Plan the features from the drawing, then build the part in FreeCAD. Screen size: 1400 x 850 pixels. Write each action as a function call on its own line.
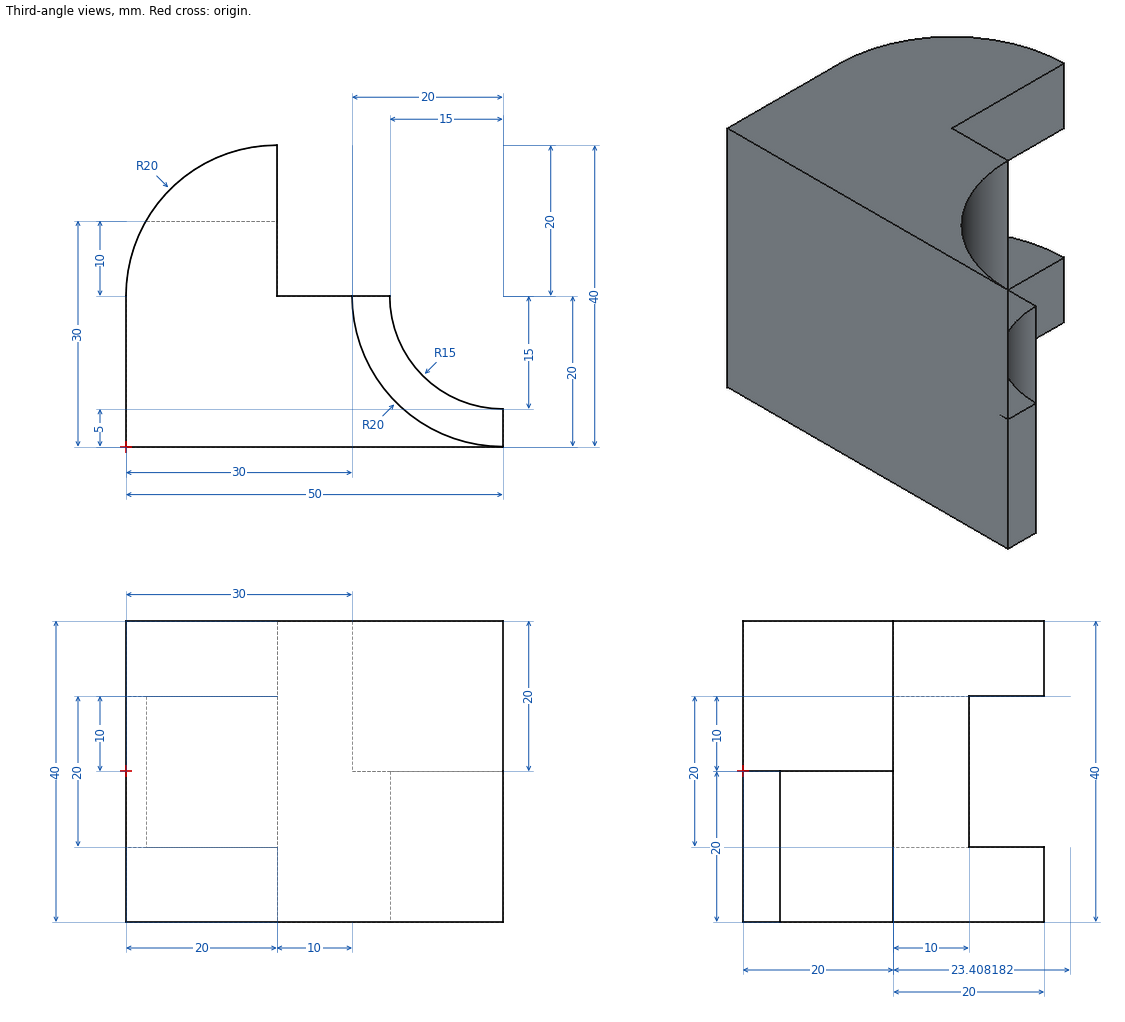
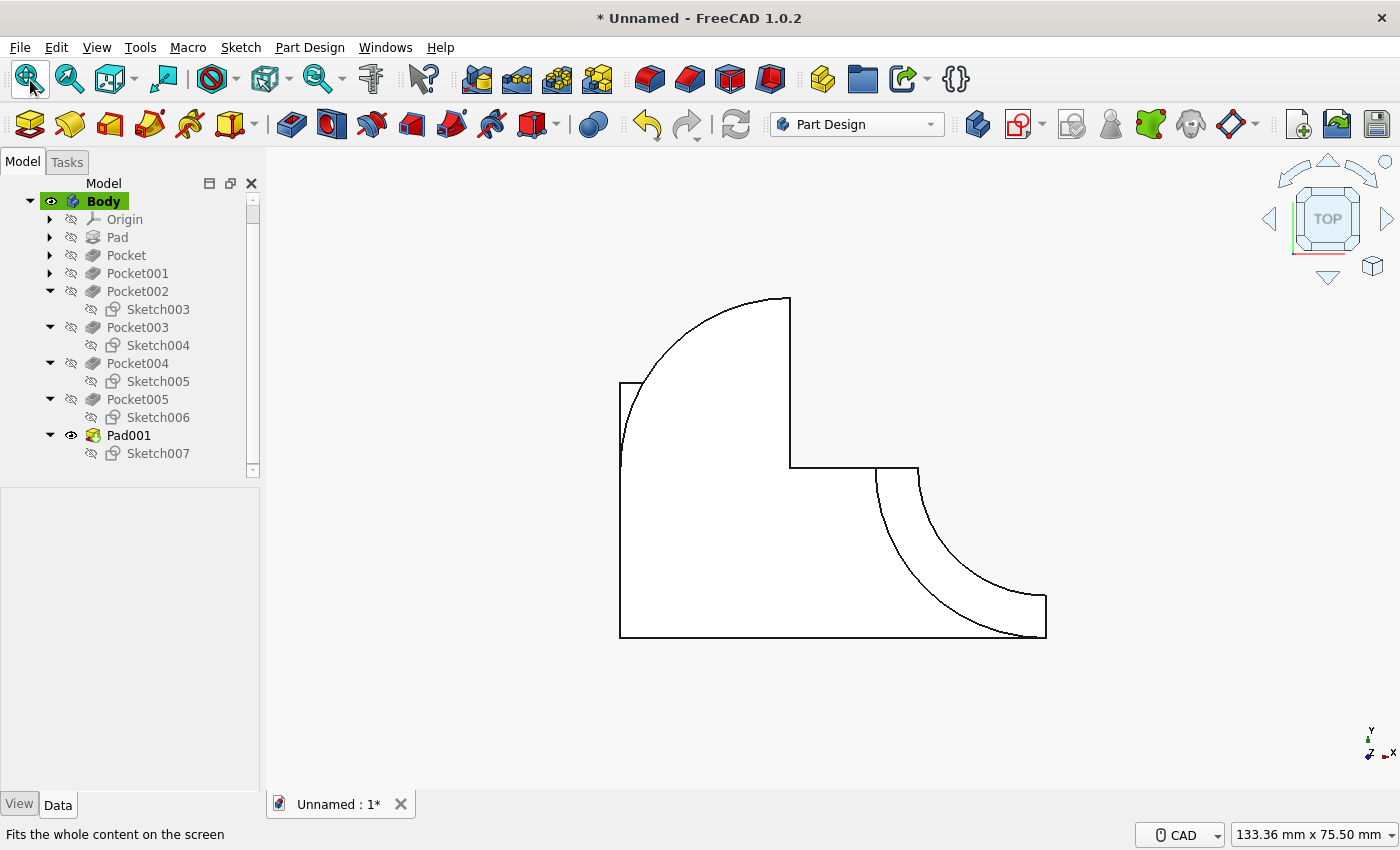
scroll(632, 388, up, 4)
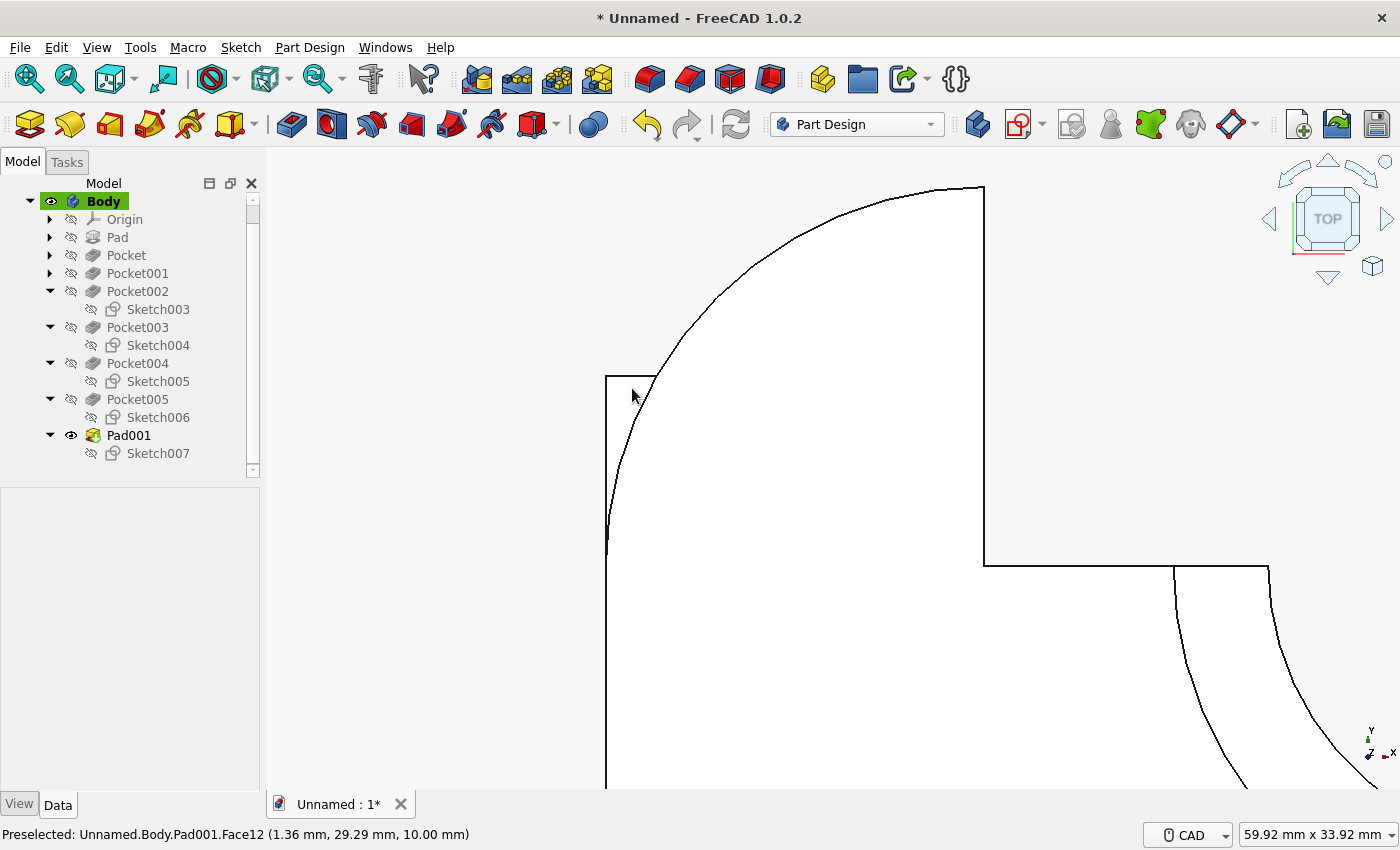
click(631, 389)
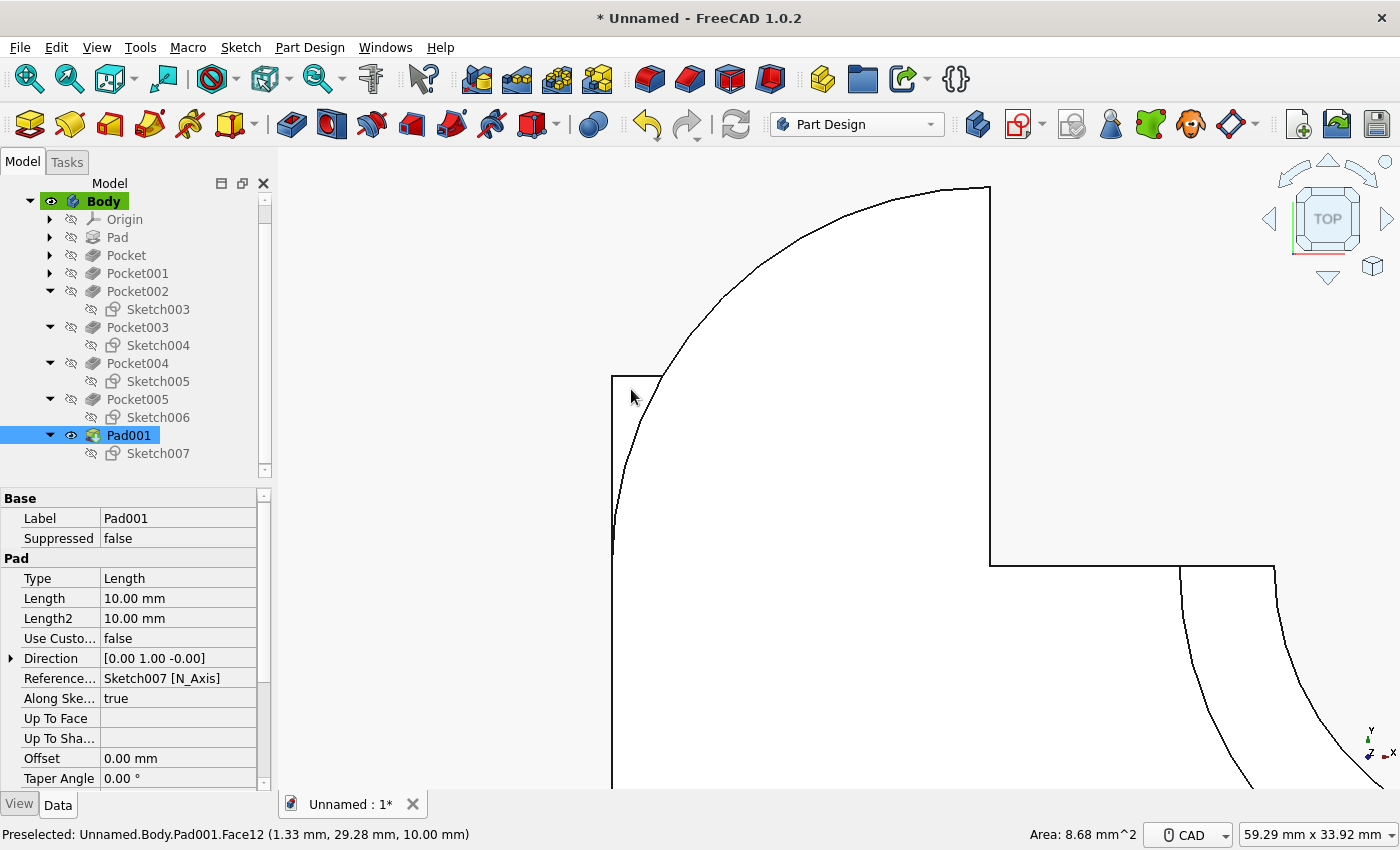
click(1018, 124)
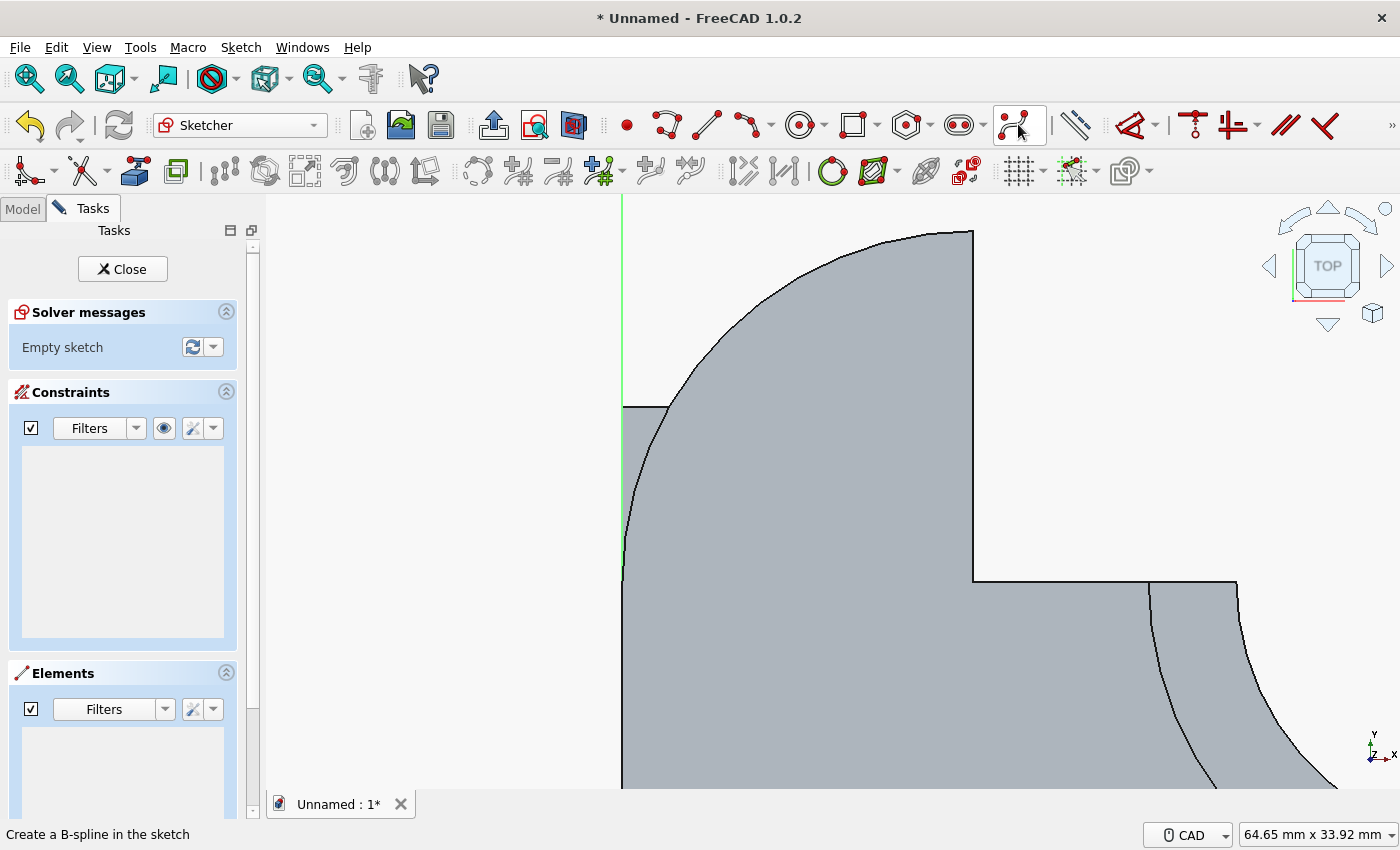
scroll(549, 496, up, 4)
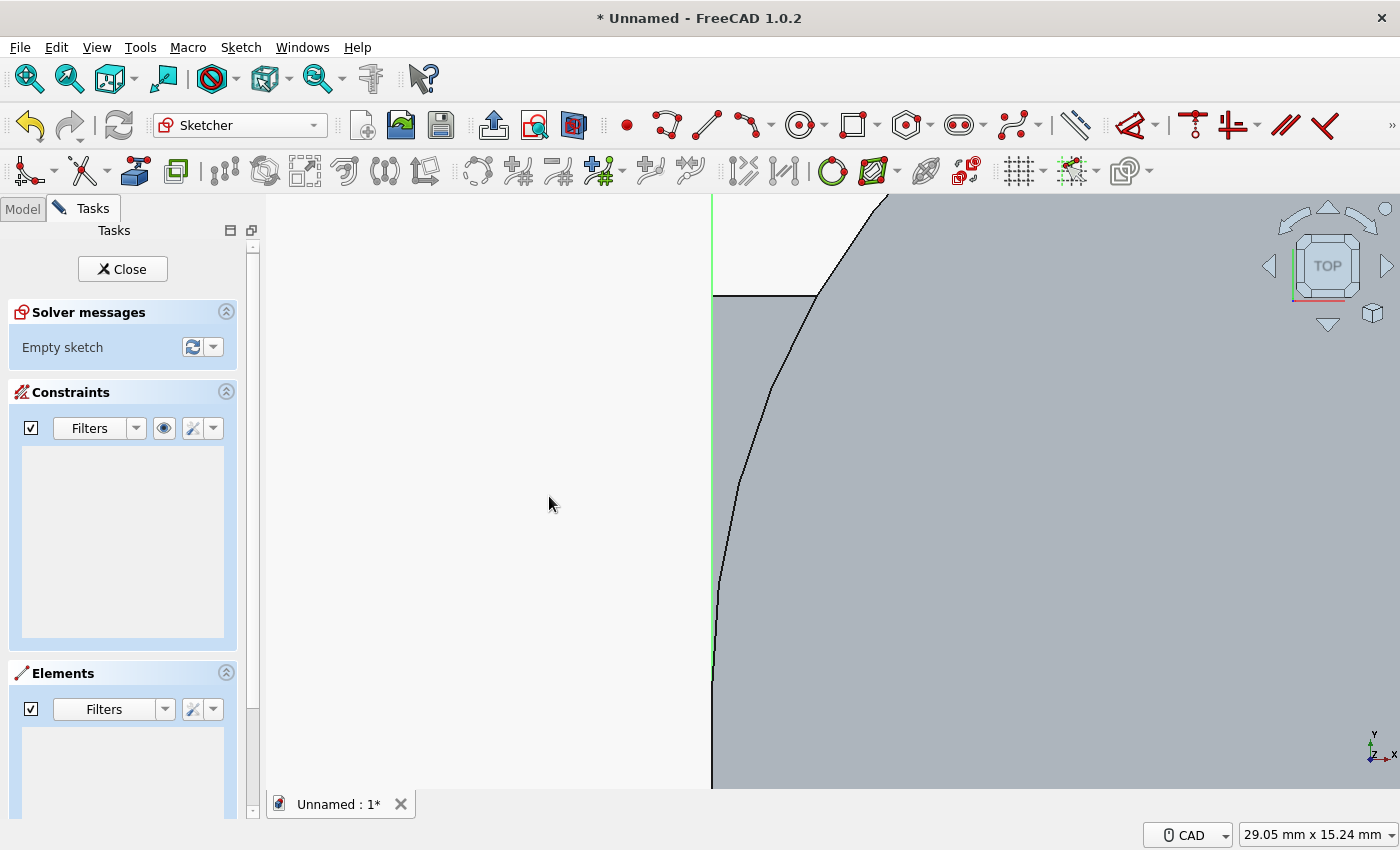
click(668, 126)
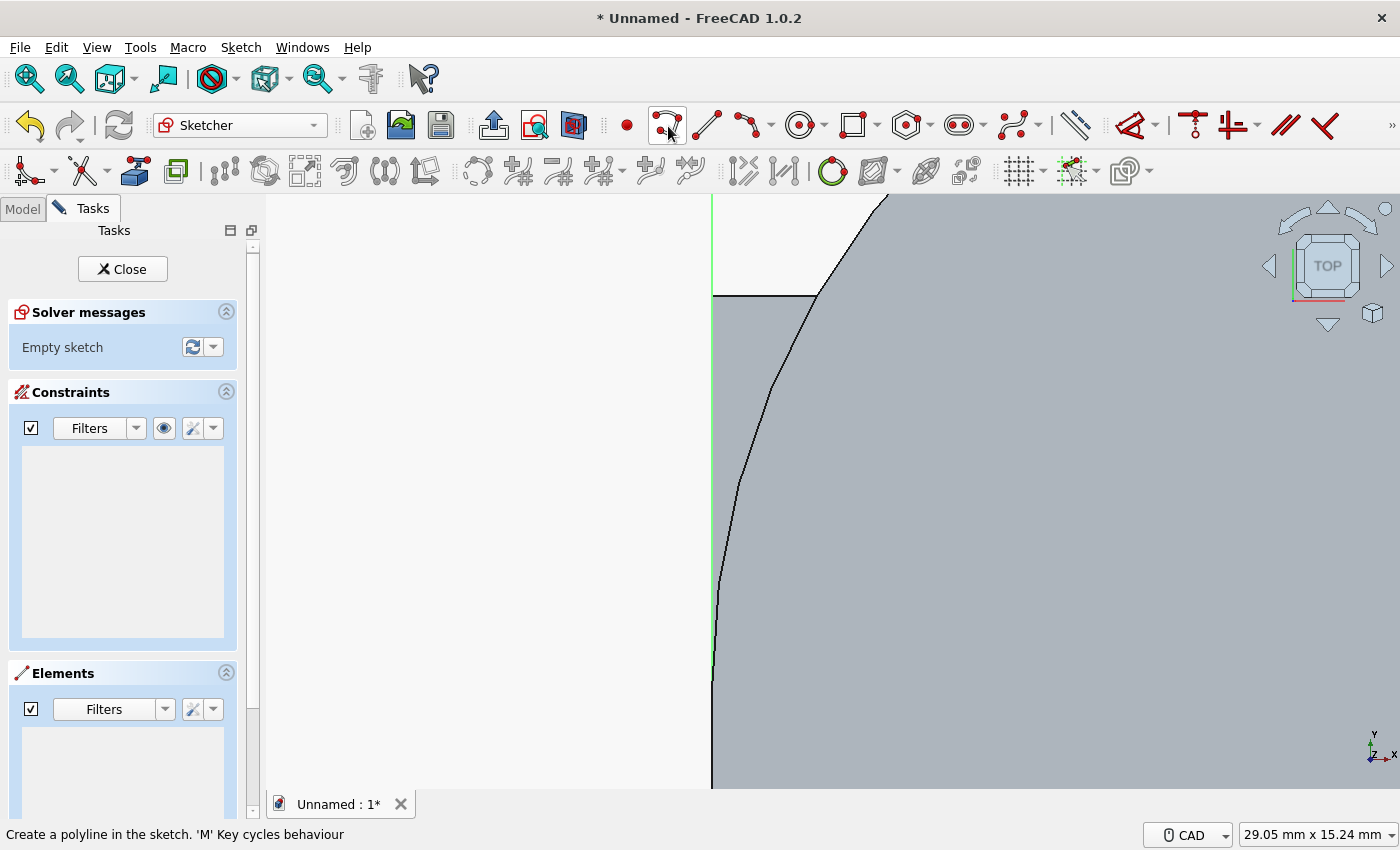
click(817, 296)
click(712, 296)
click(721, 687)
right_click(721, 687)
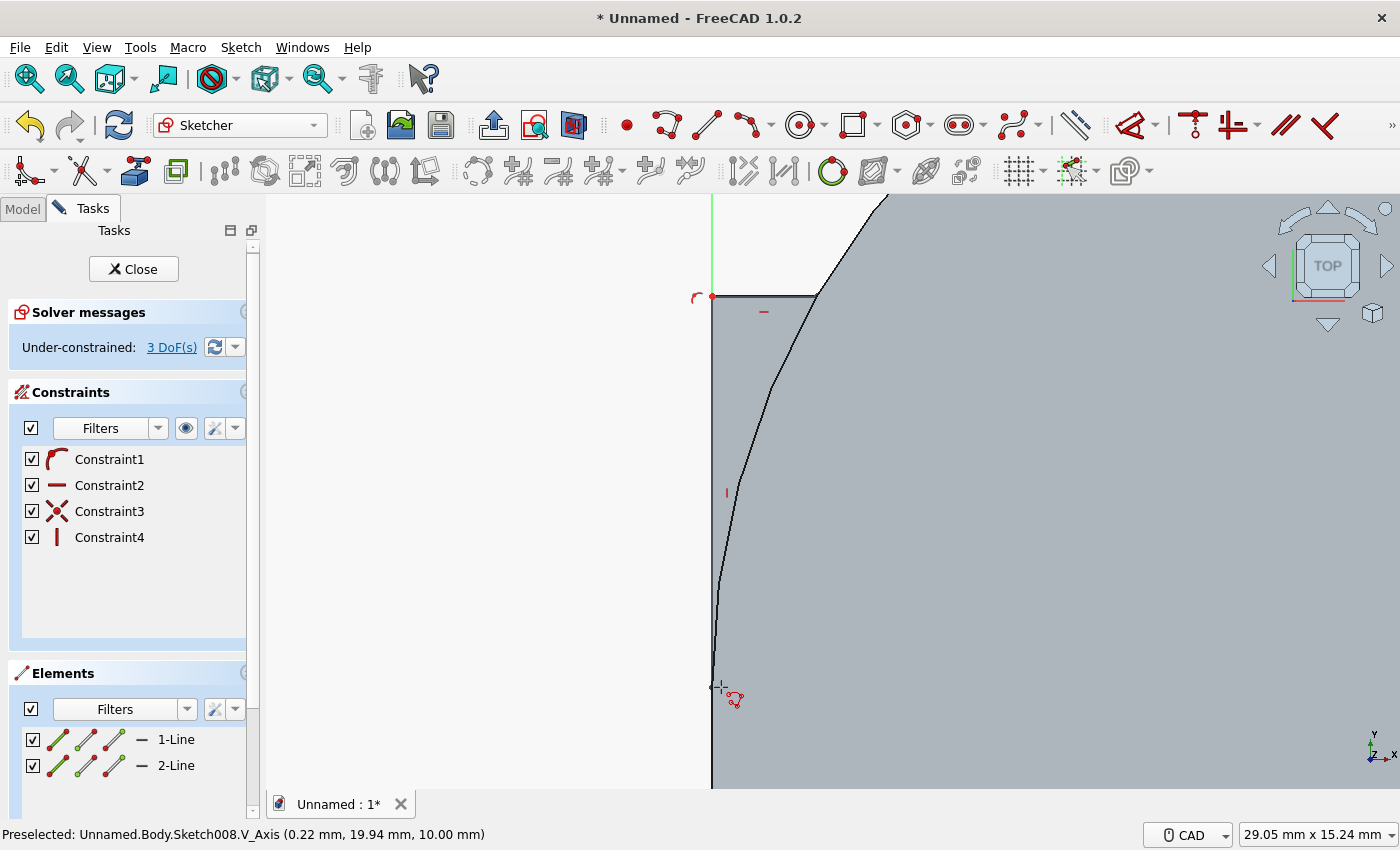
click(748, 126)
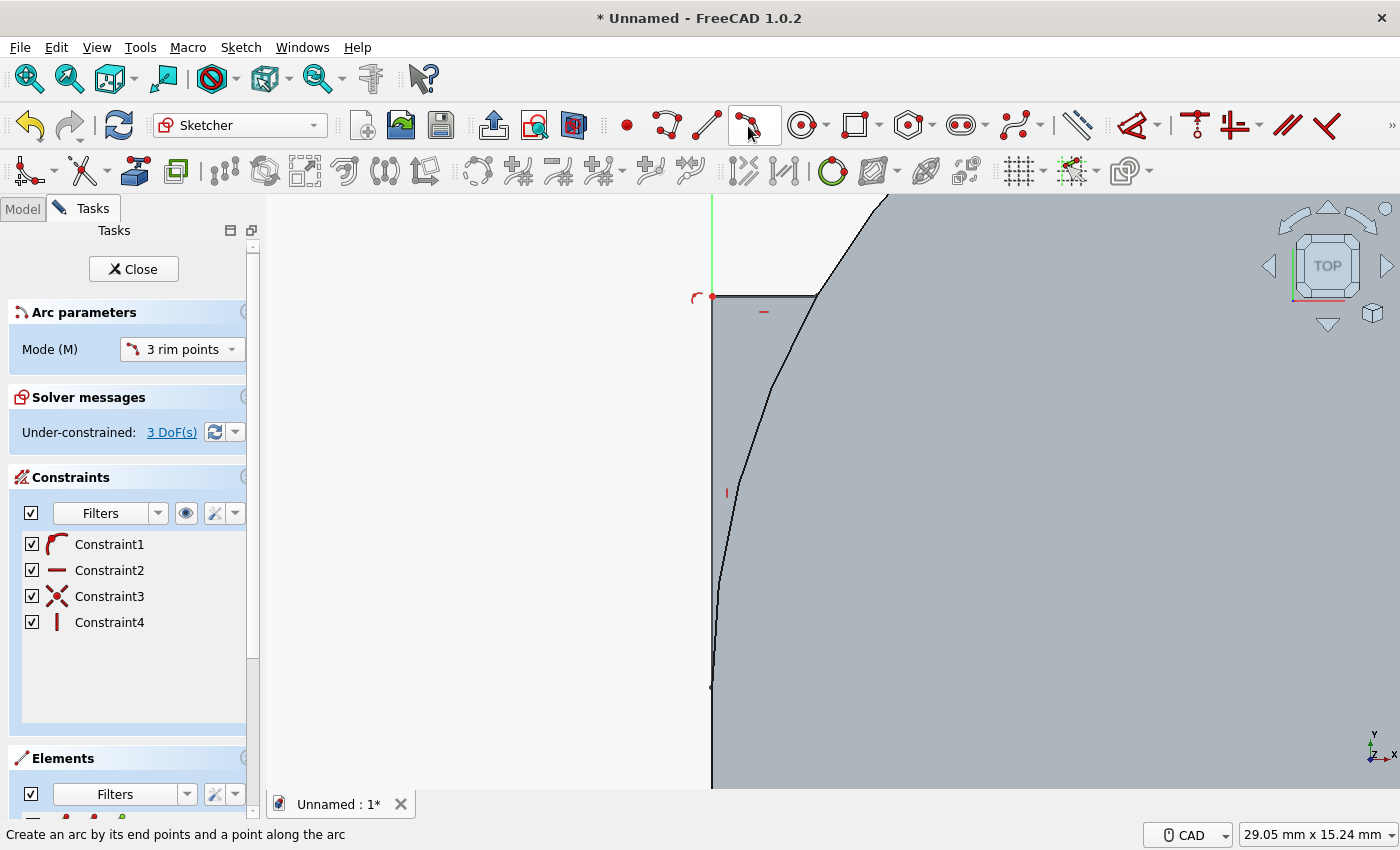
click(712, 688)
click(817, 297)
click(739, 485)
key(Escape)